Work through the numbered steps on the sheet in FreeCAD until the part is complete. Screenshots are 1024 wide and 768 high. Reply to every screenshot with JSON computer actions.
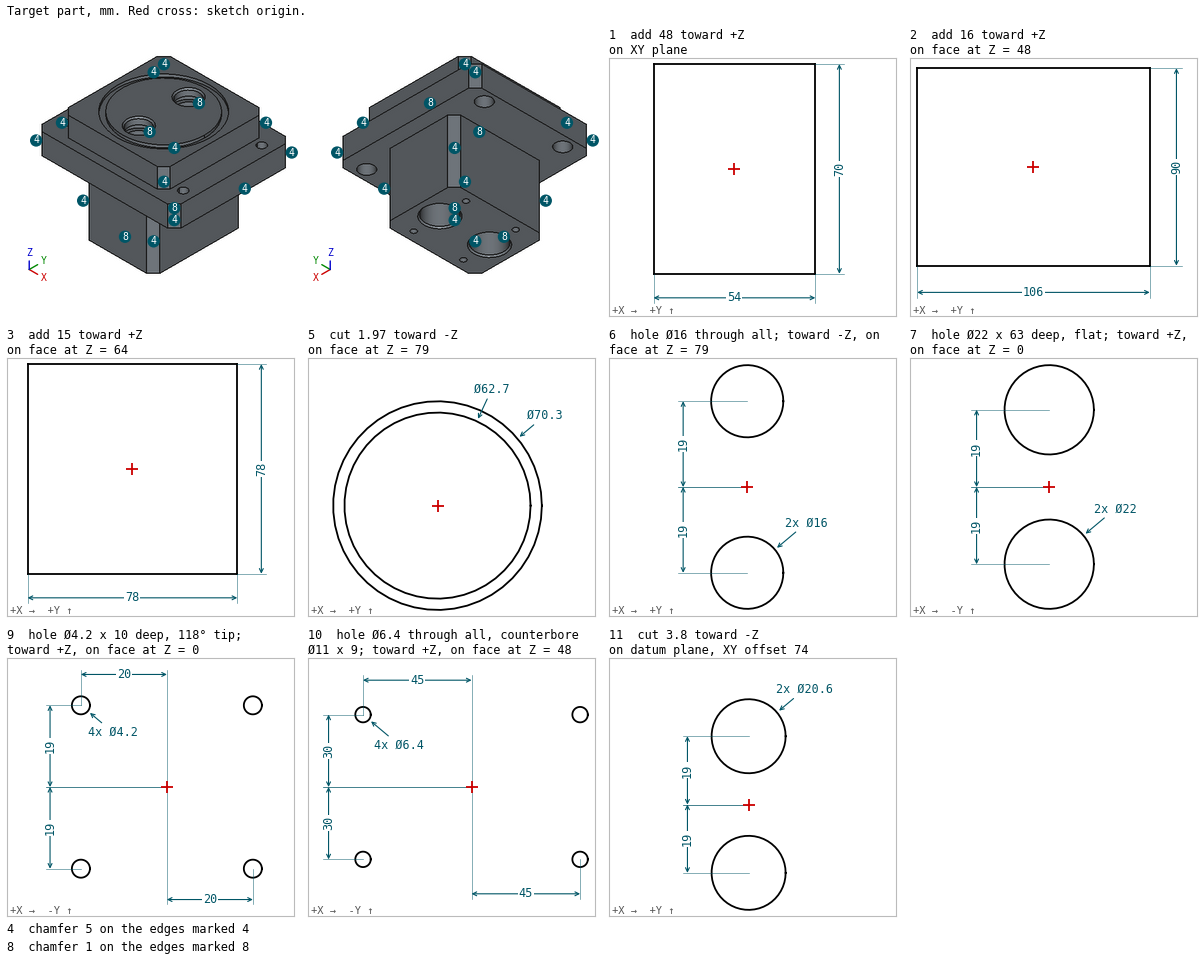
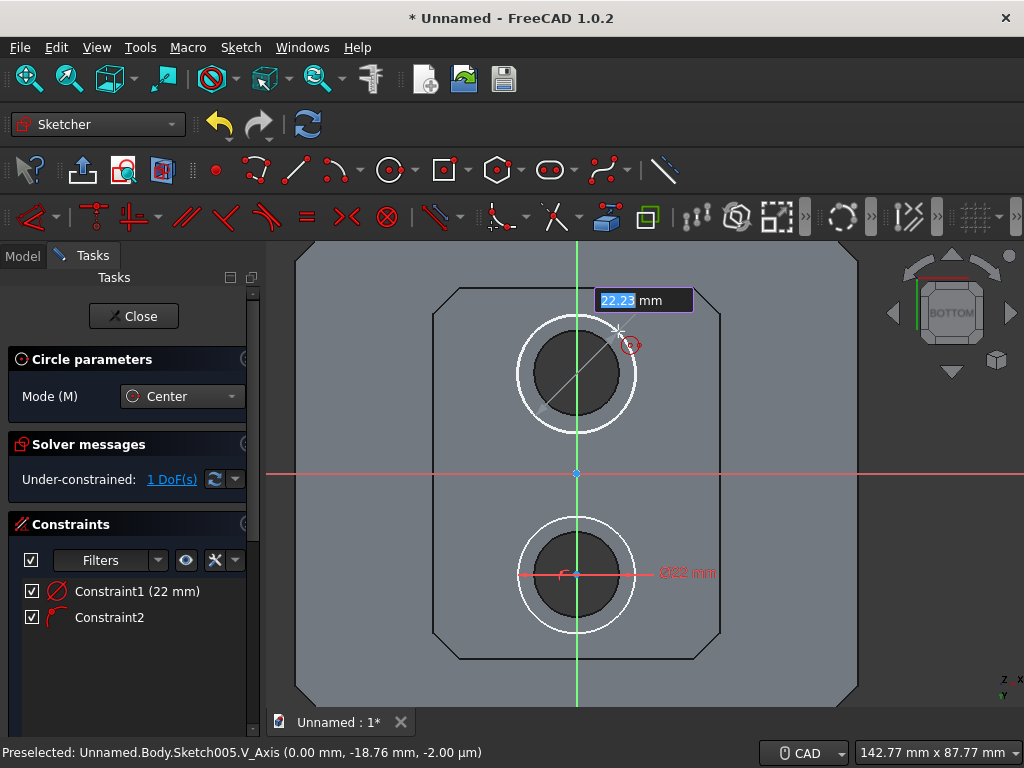
{"action": "type", "text": "22"}
{"action": "key", "text": "Return"}
{"action": "key", "text": "Escape"}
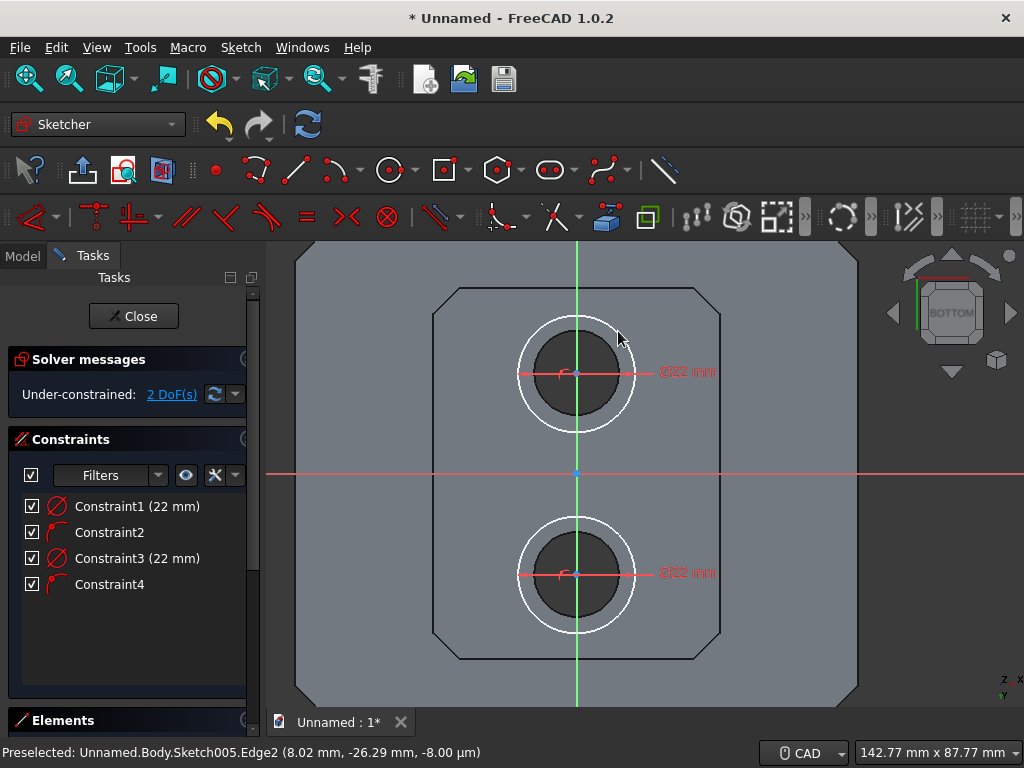
{"action": "left_click", "coordinate": [32, 218]}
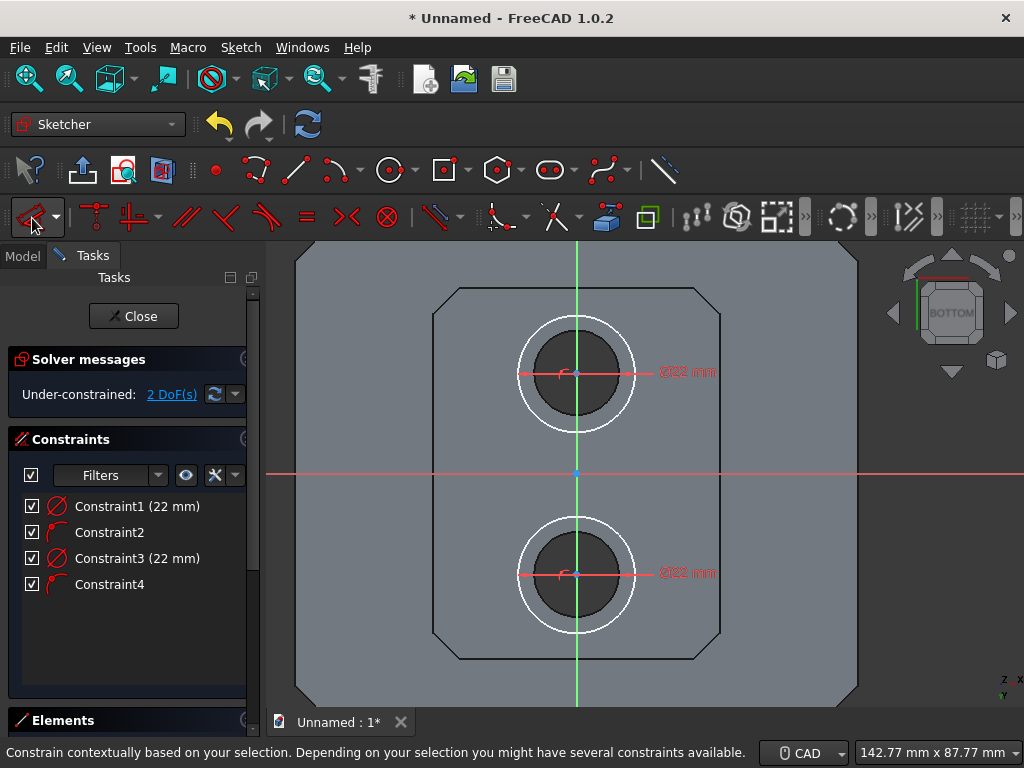
{"action": "left_click", "coordinate": [577, 575]}
{"action": "left_click", "coordinate": [611, 501]}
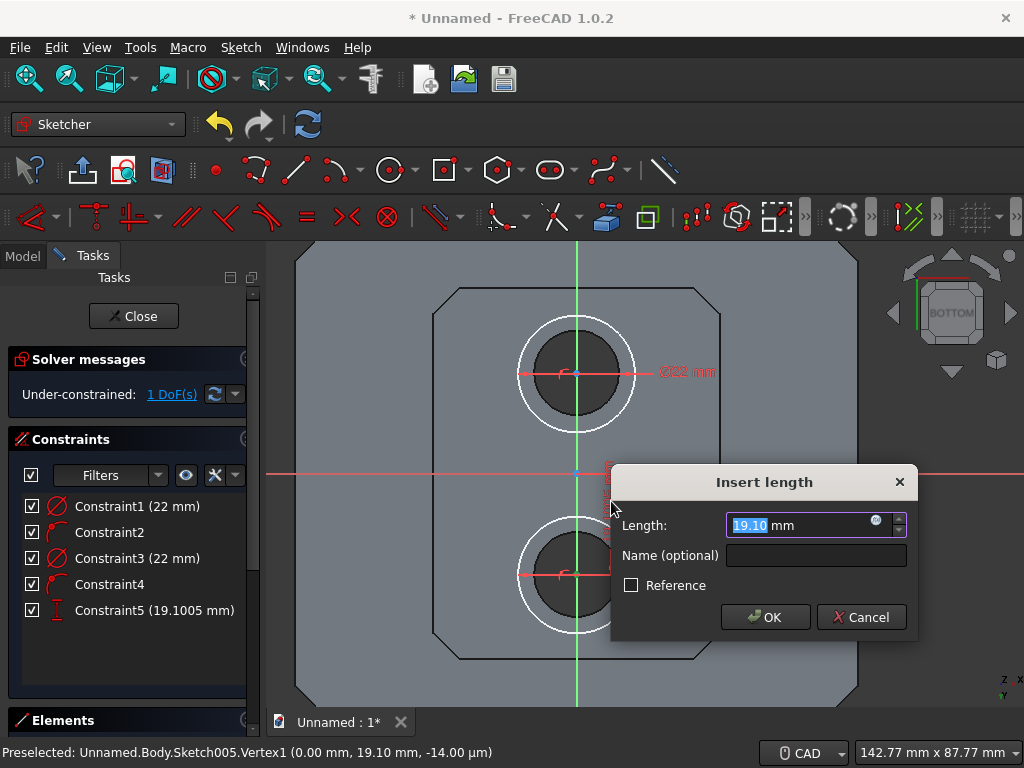
{"action": "type", "text": "19"}
{"action": "key", "text": "Return"}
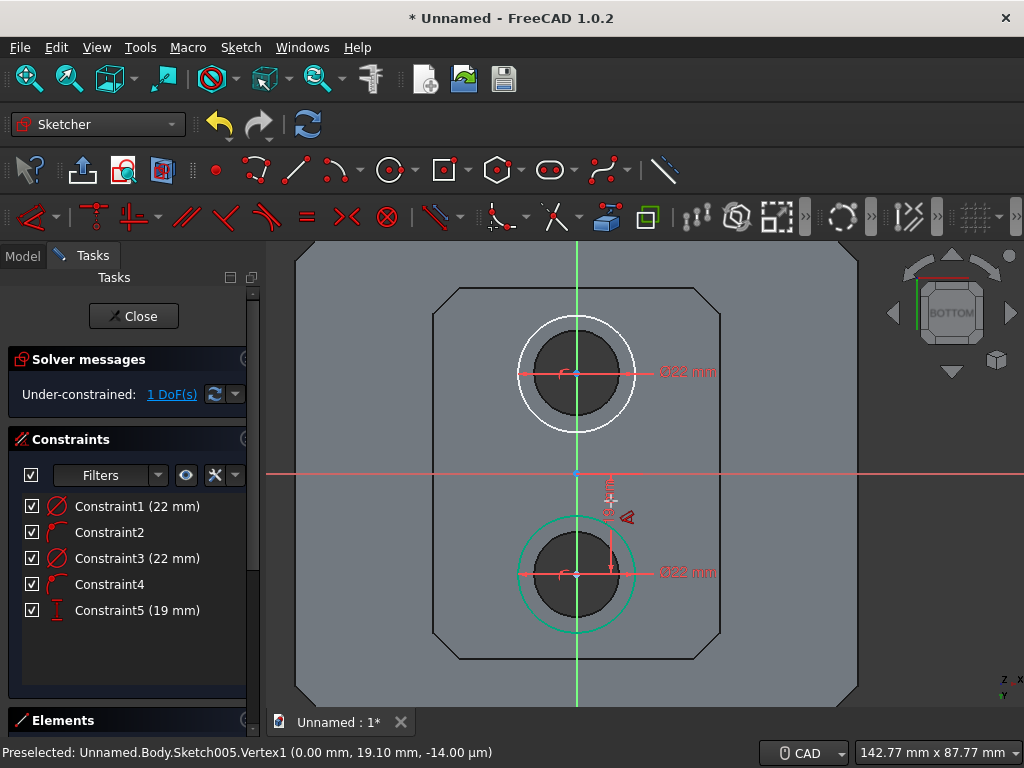
{"action": "left_click", "coordinate": [577, 374]}
{"action": "left_click", "coordinate": [611, 401]}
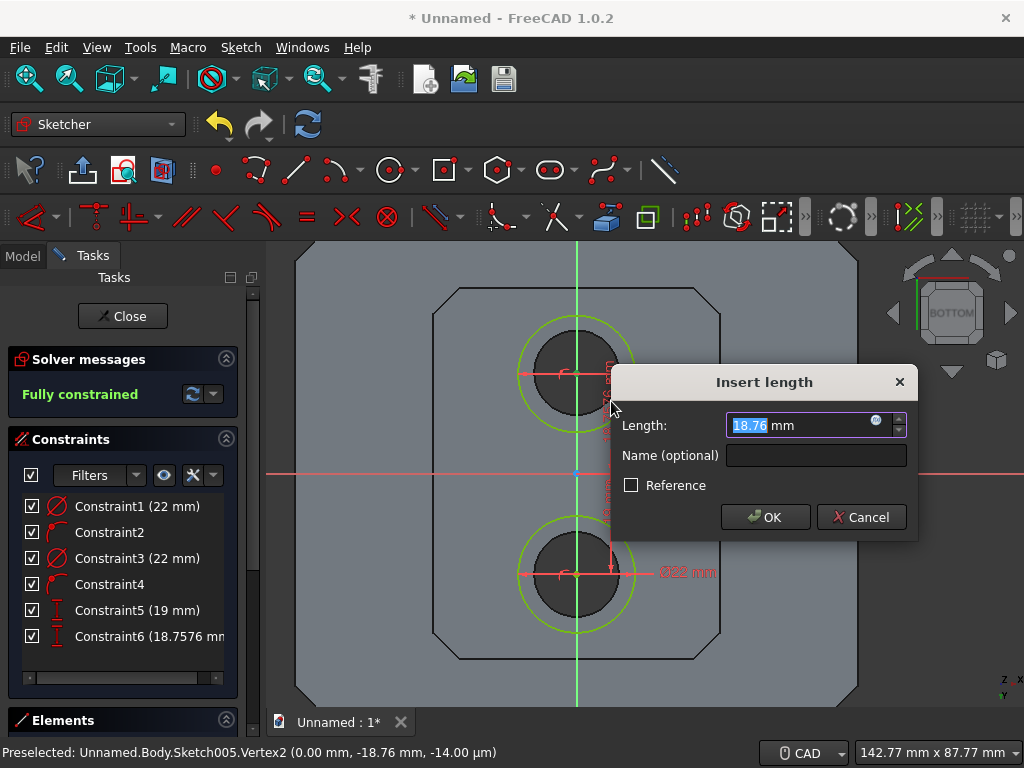
{"action": "type", "text": "19"}
{"action": "key", "text": "Return"}
{"action": "key", "text": "Escape"}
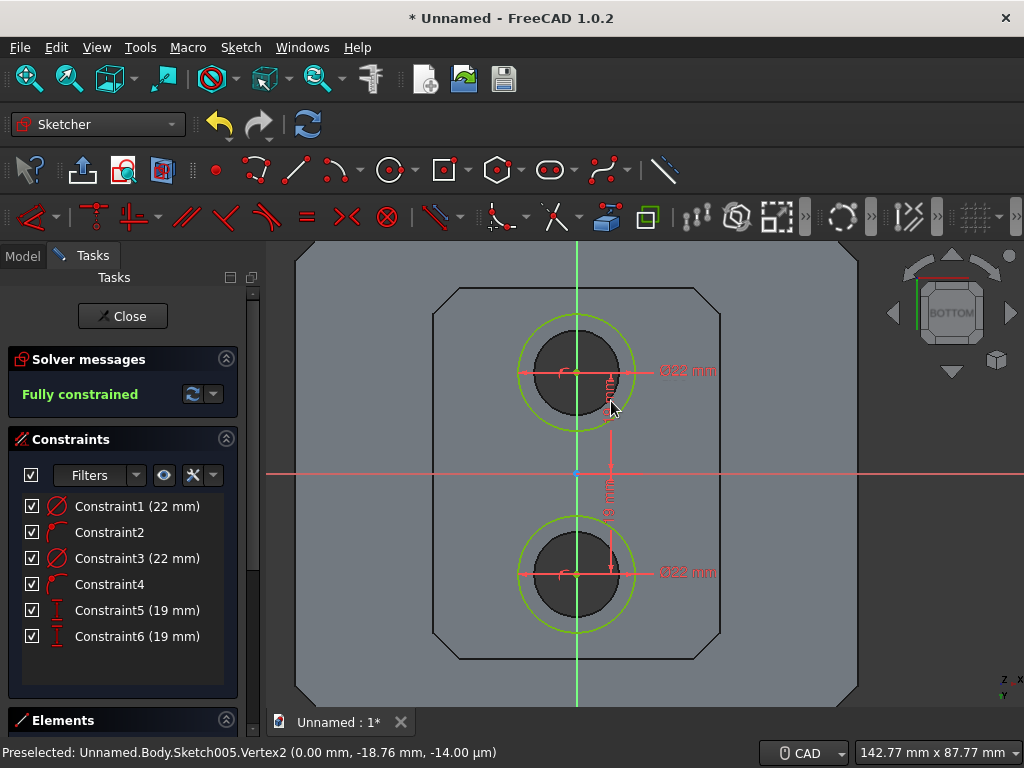
{"action": "left_click", "coordinate": [123, 316]}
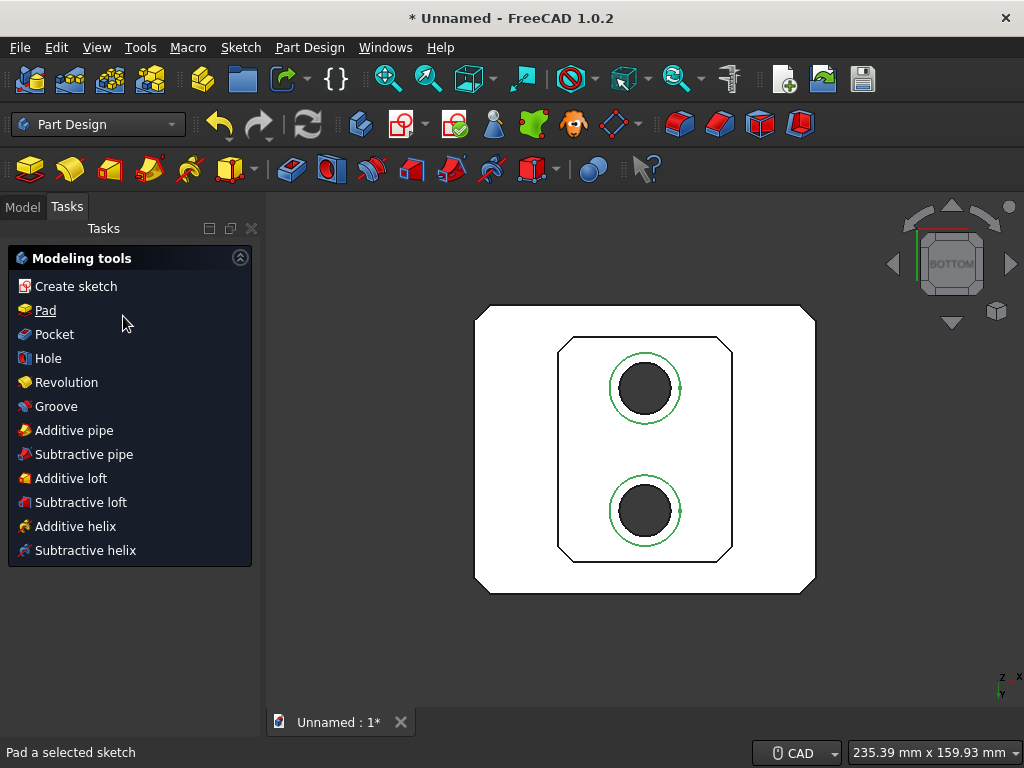
{"action": "left_click", "coordinate": [332, 170]}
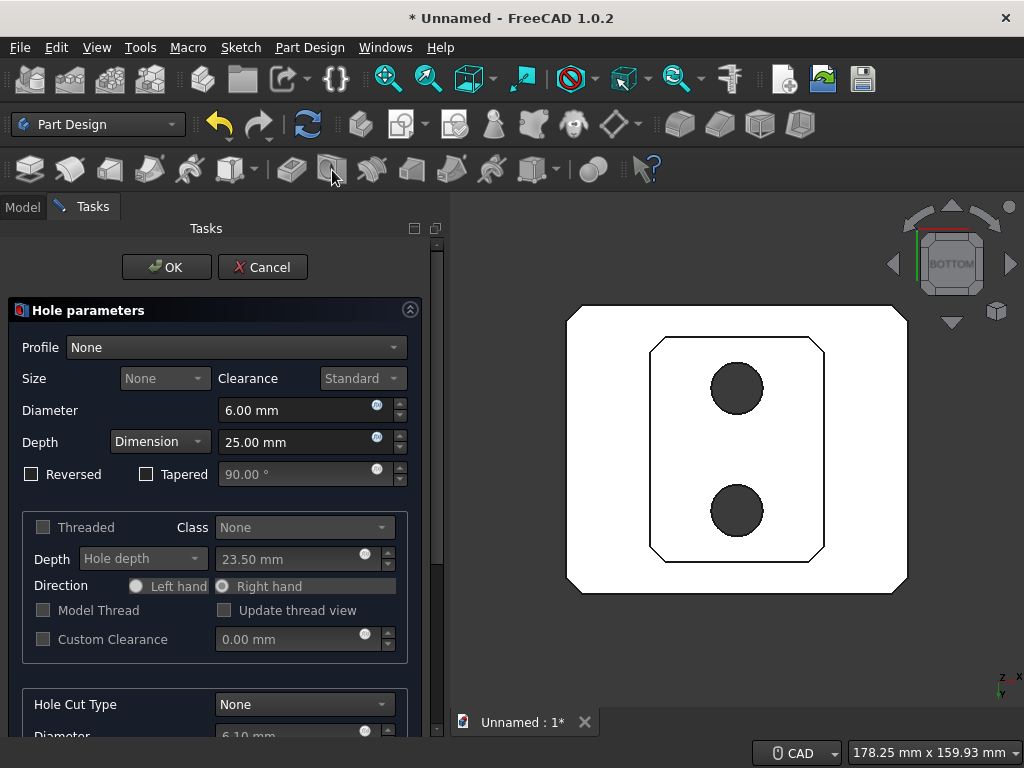
{"action": "triple_click", "coordinate": [305, 410]}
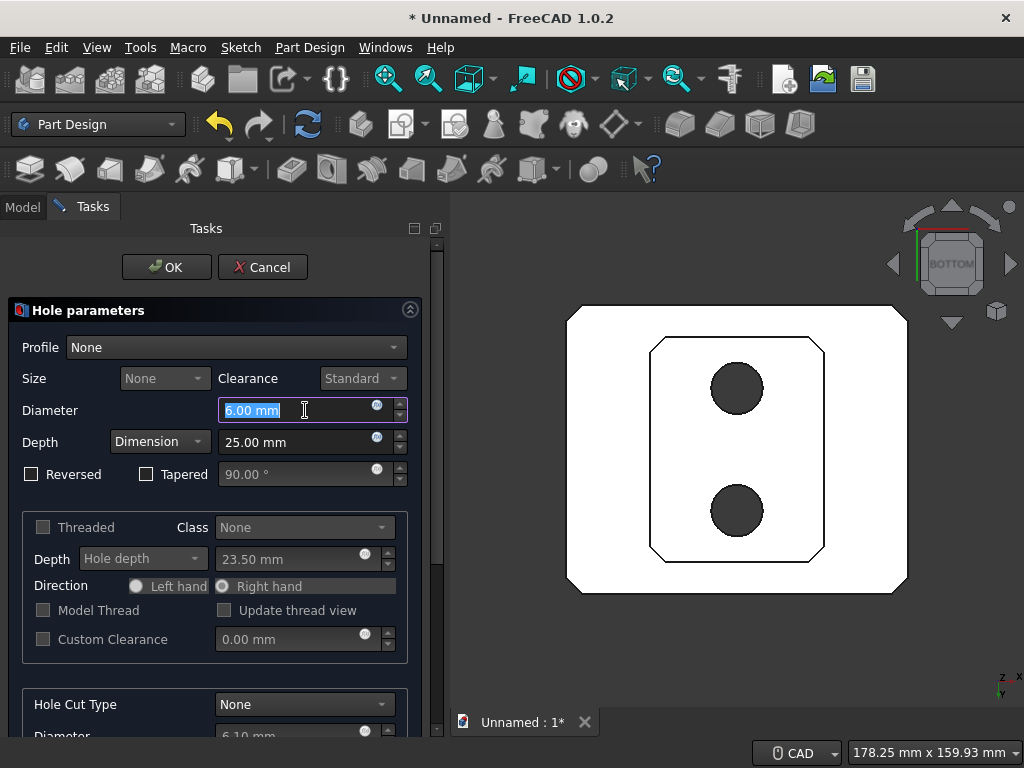
{"action": "type", "text": "22"}
{"action": "key", "text": "Tab"}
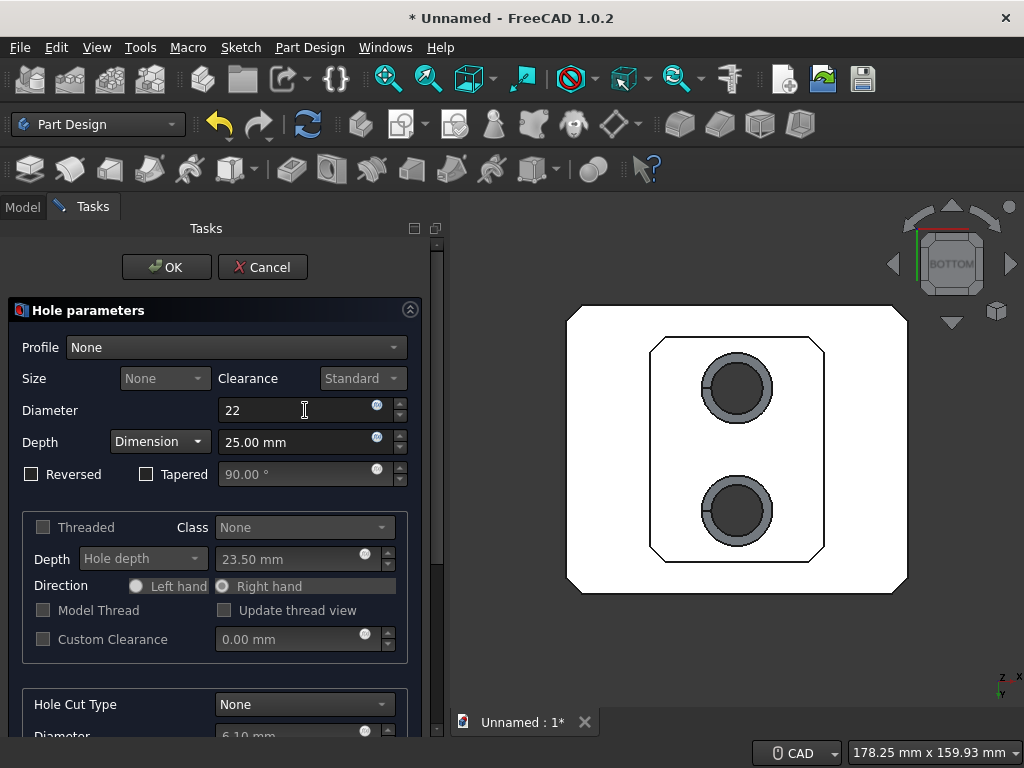
{"action": "triple_click", "coordinate": [305, 442]}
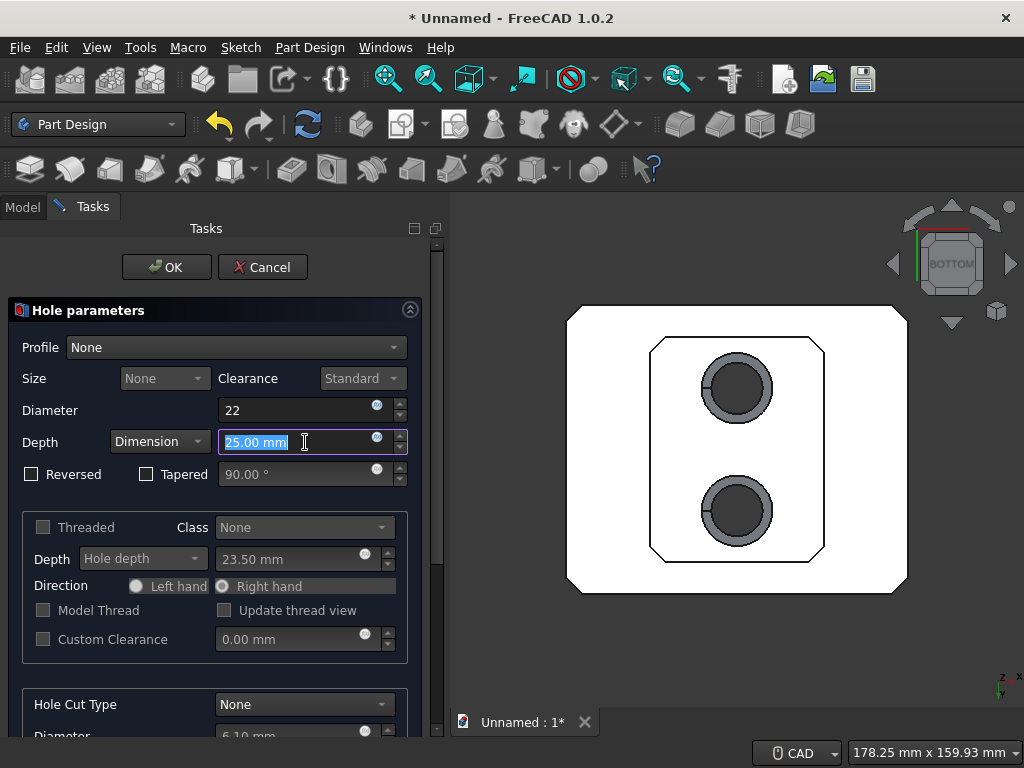
{"action": "type", "text": "63"}
{"action": "key", "text": "Tab"}